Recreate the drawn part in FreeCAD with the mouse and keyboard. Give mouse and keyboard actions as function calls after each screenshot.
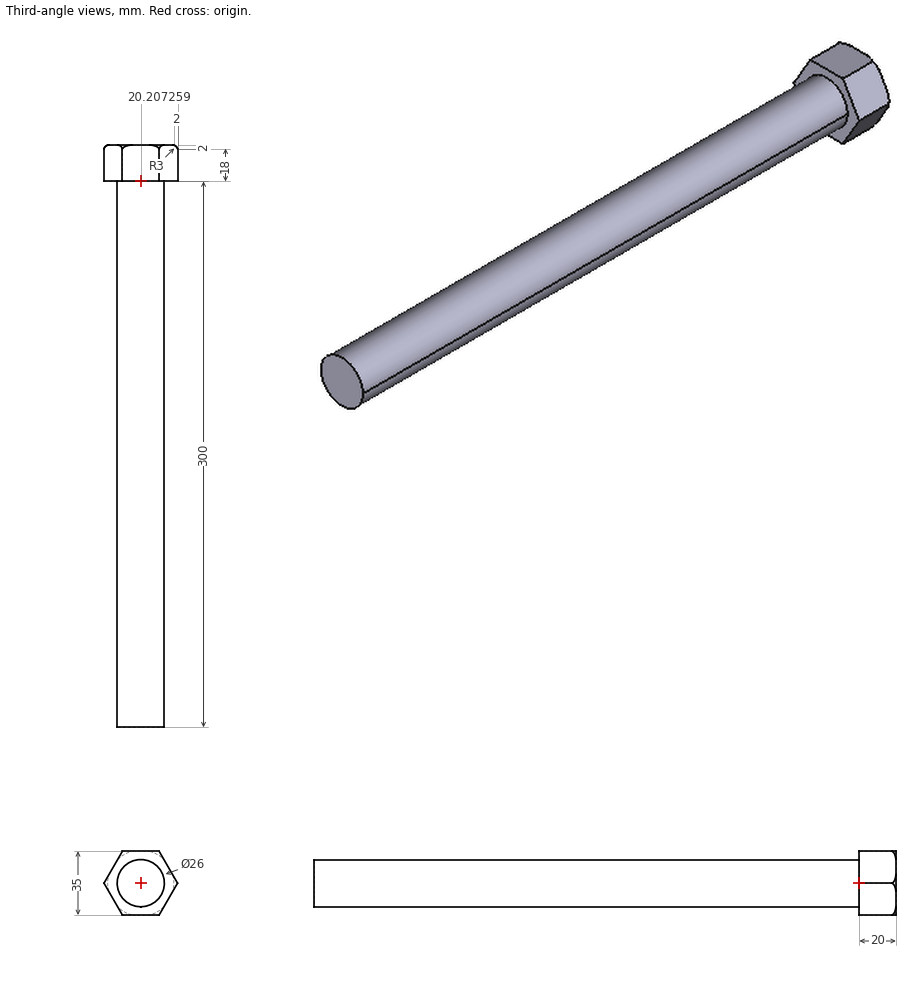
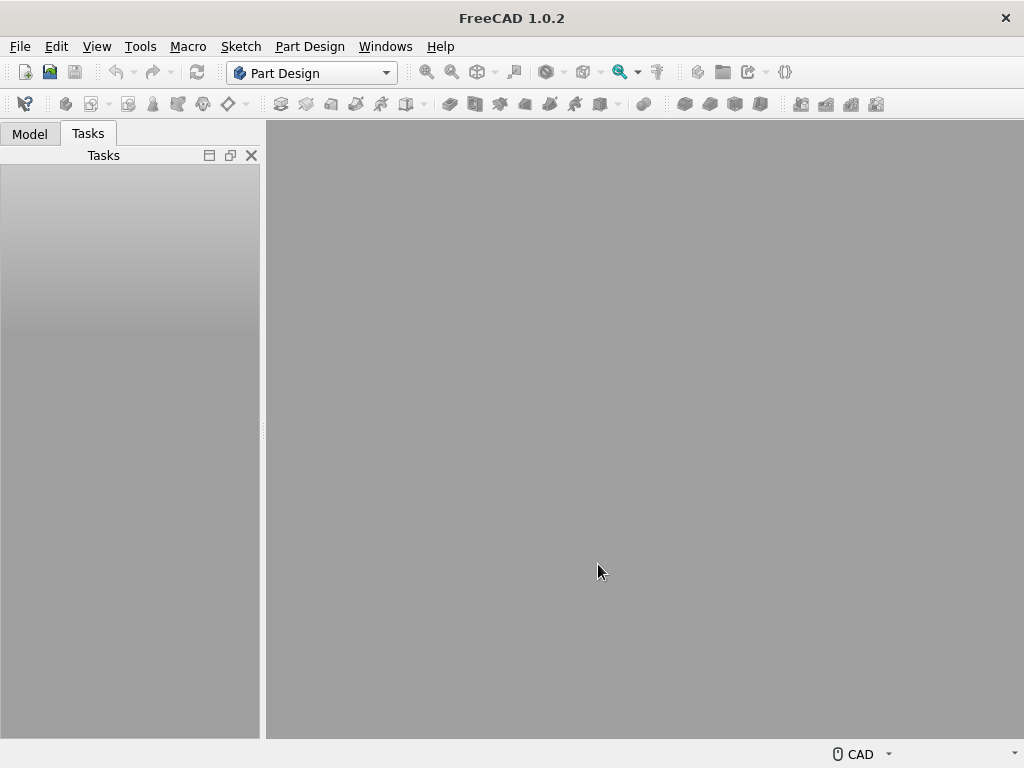
click(25, 72)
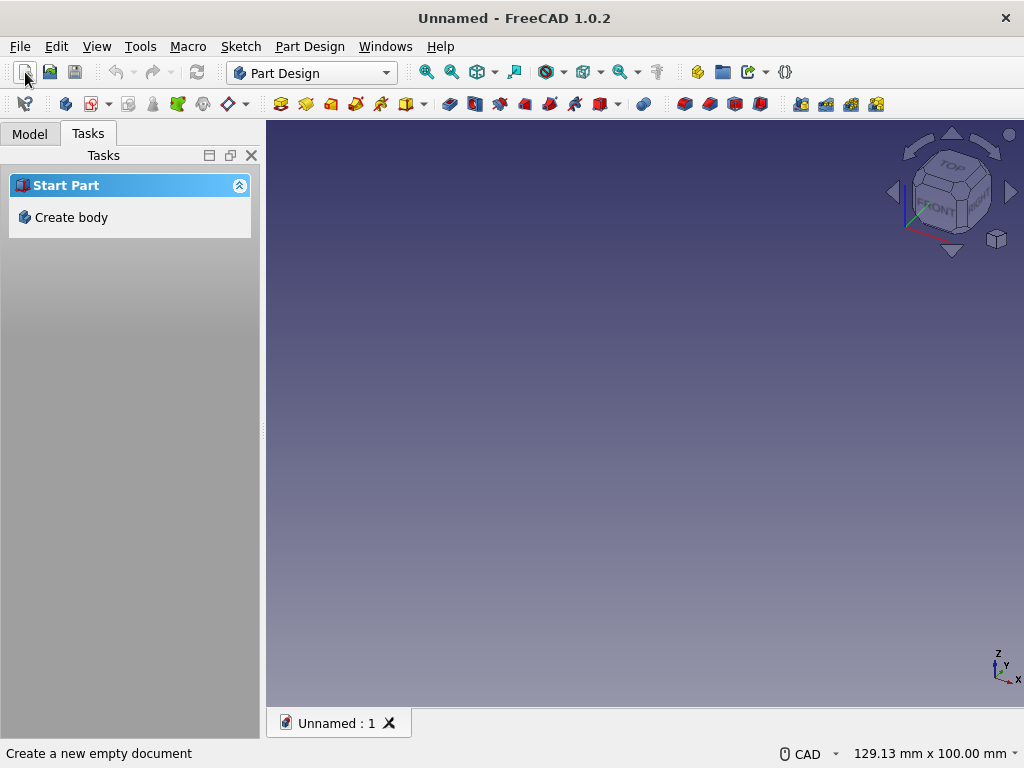
click(90, 104)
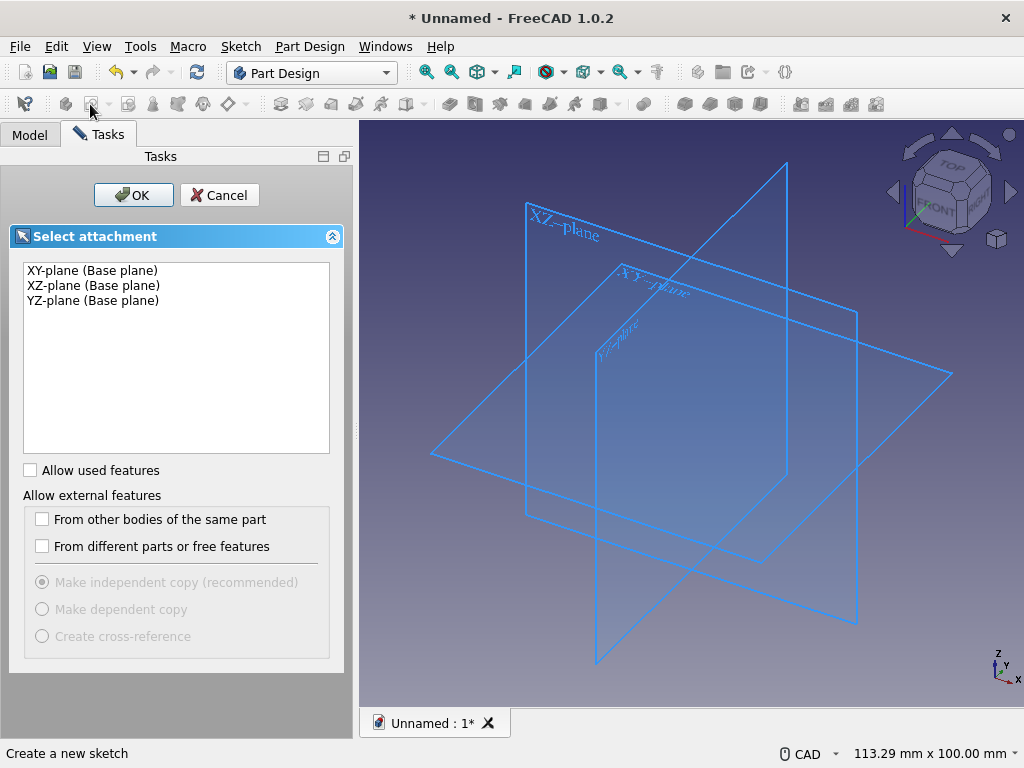
click(84, 286)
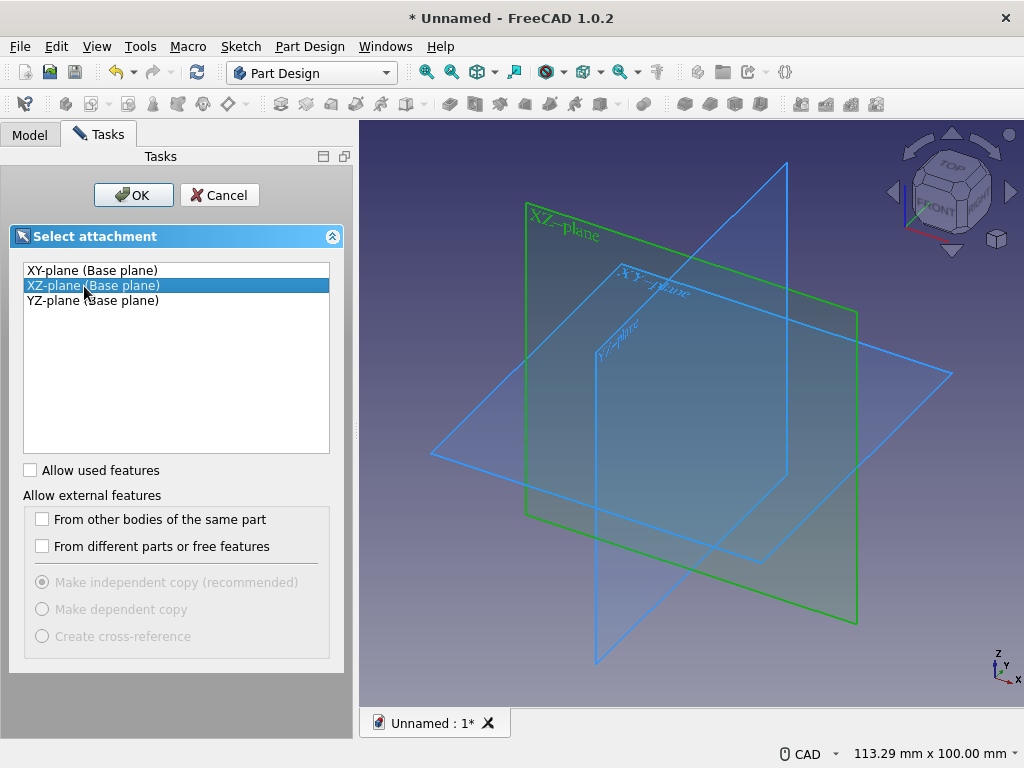
click(134, 195)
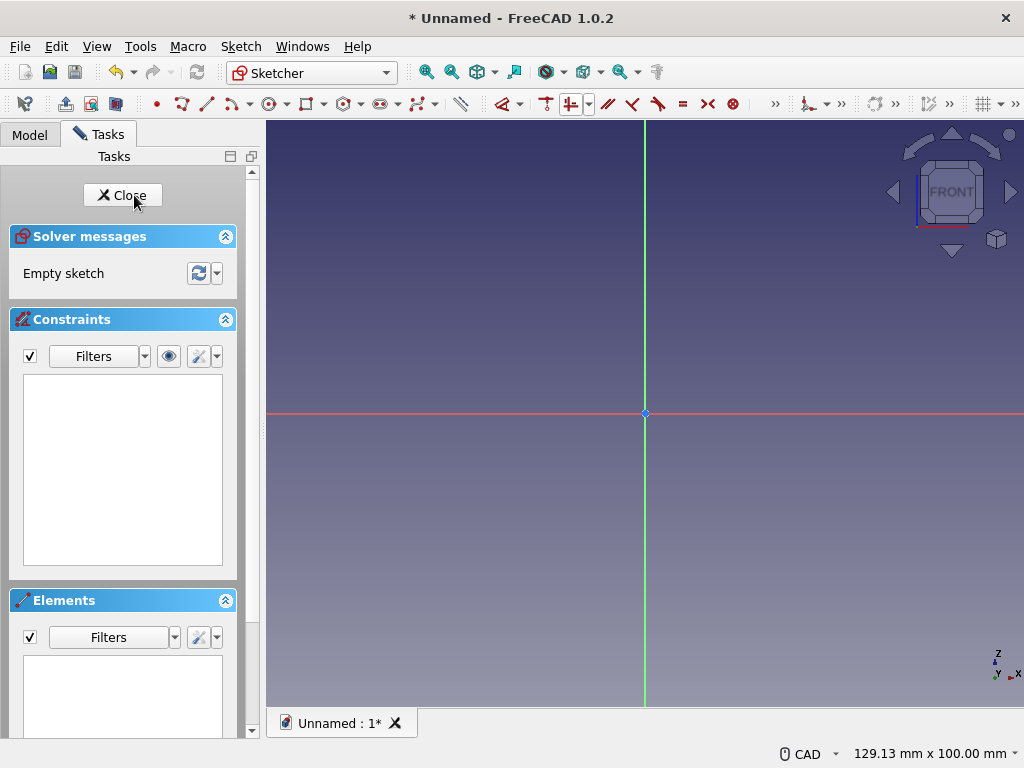
scroll(728, 414, up, 3)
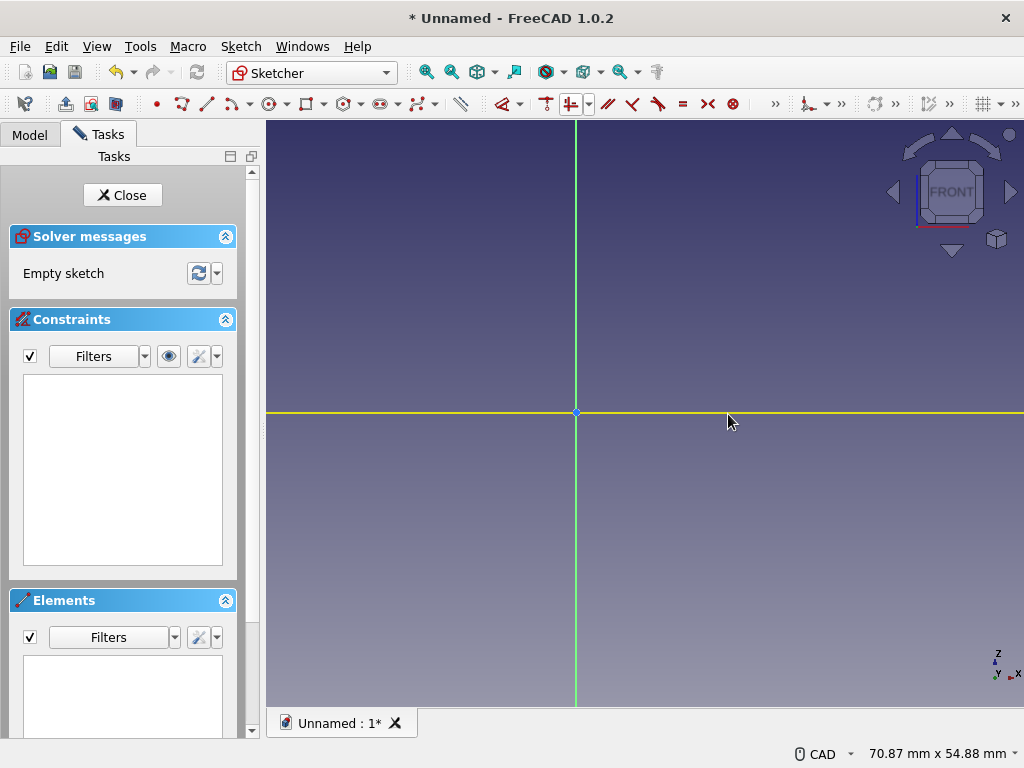
key(g)
key(p)
key(6)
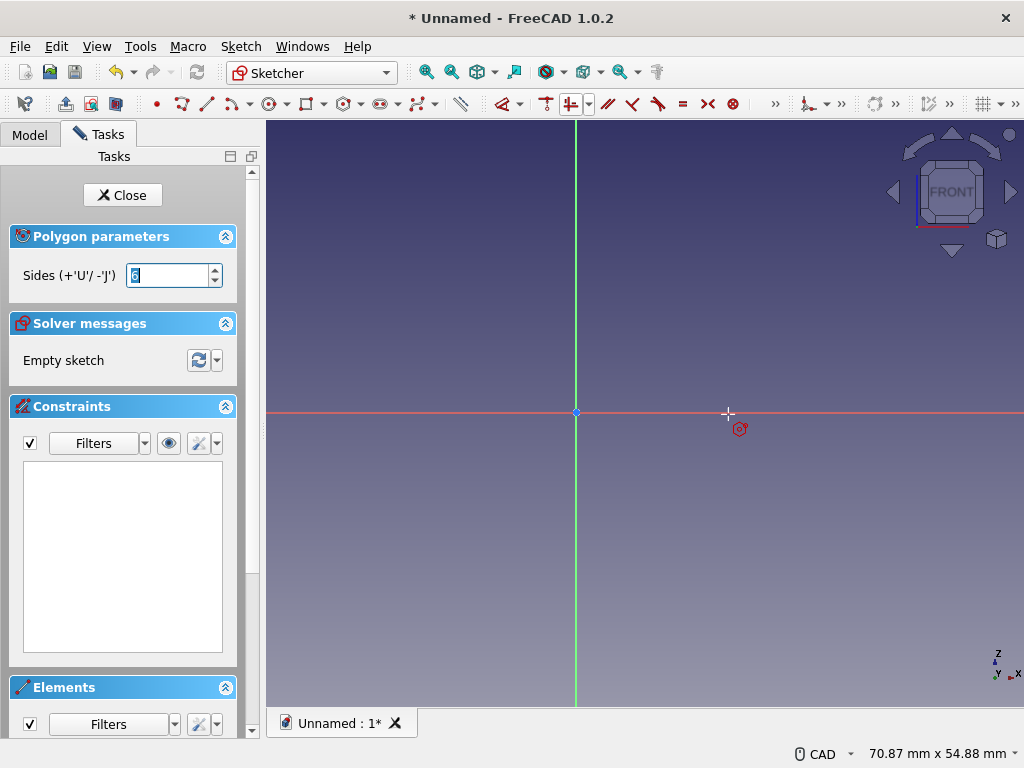
click(576, 413)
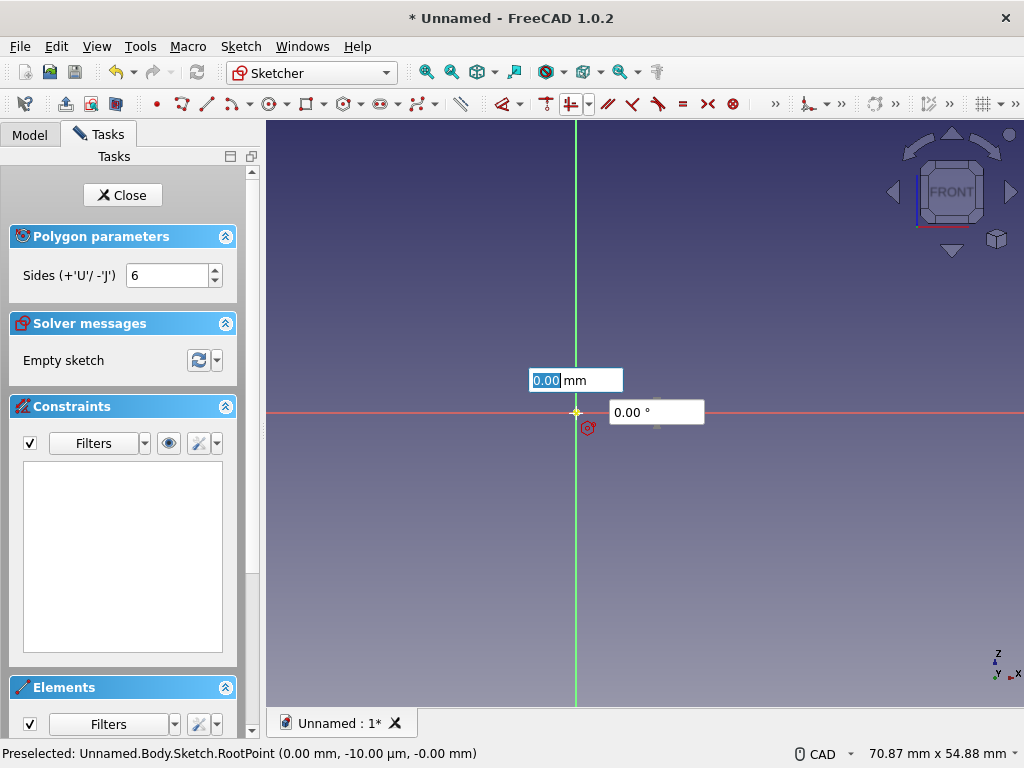
click(792, 413)
right_click(792, 413)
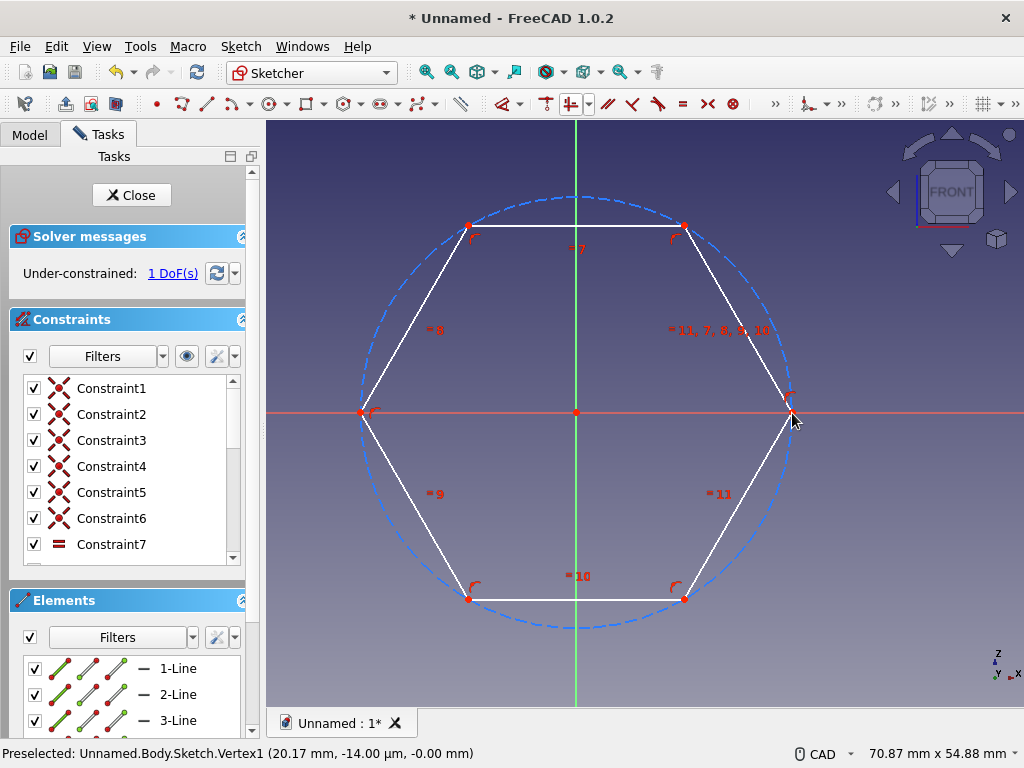
key(d)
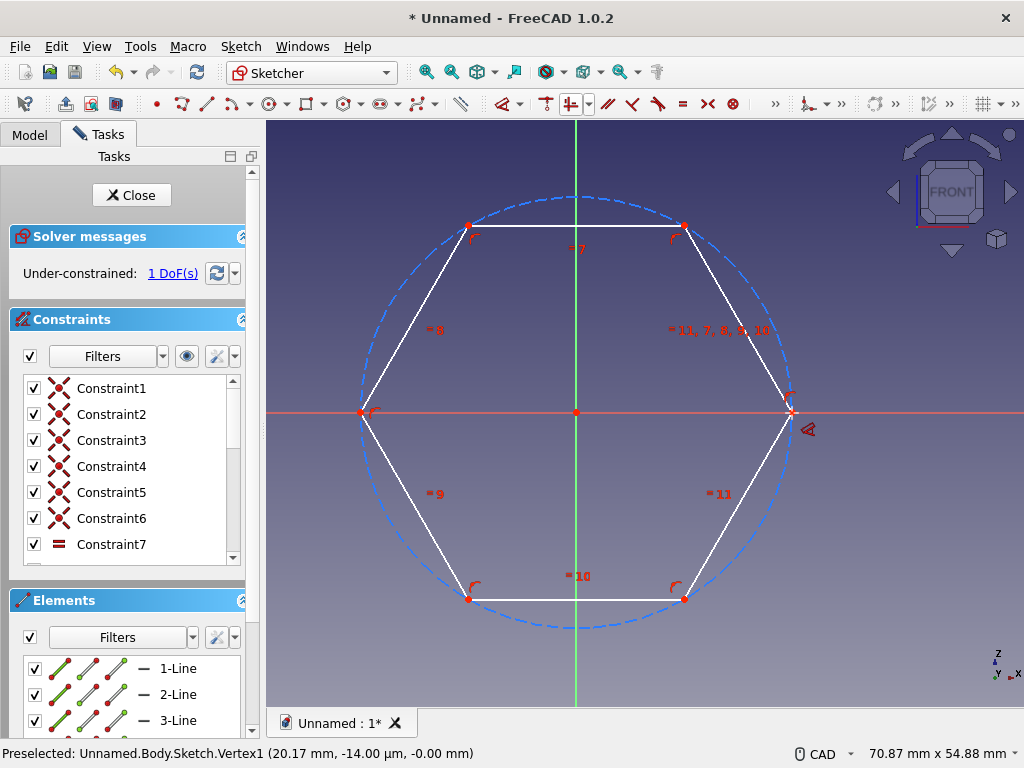
click(468, 600)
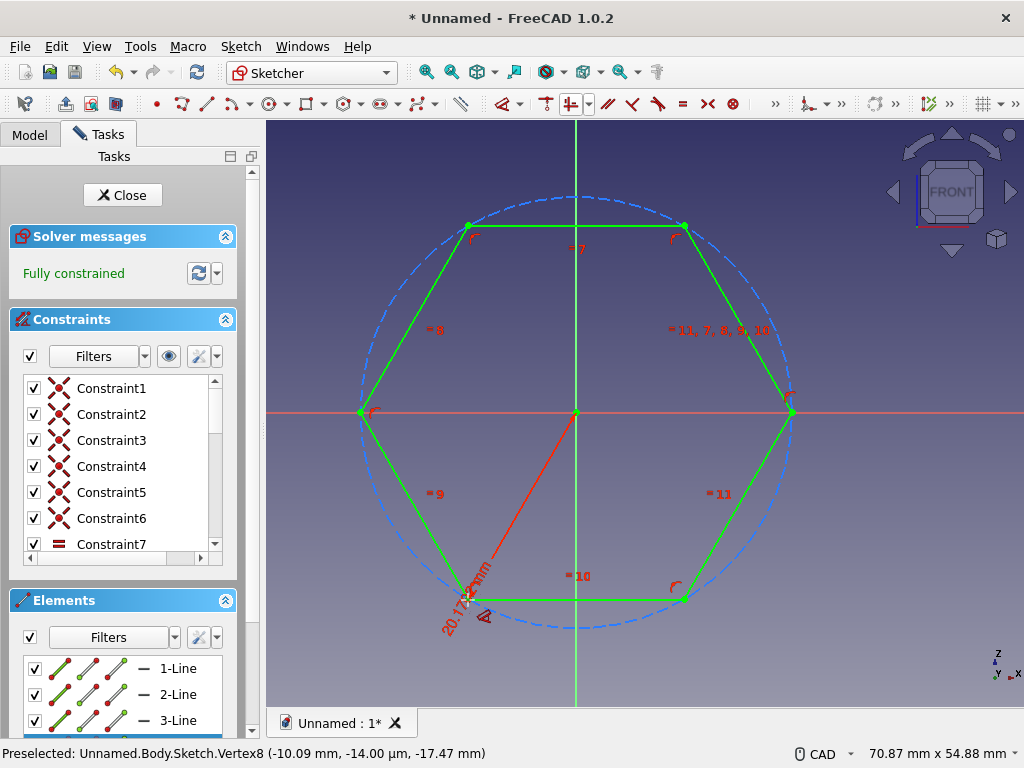
click(684, 226)
click(718, 327)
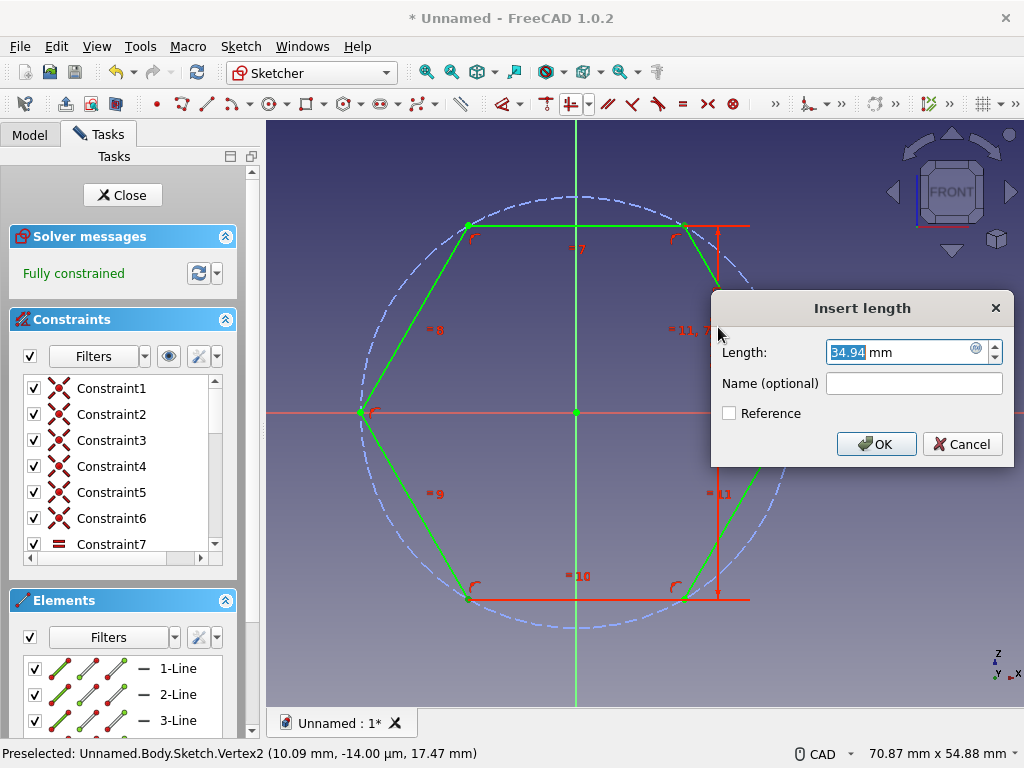
text(35)
key(Return)
key(Escape)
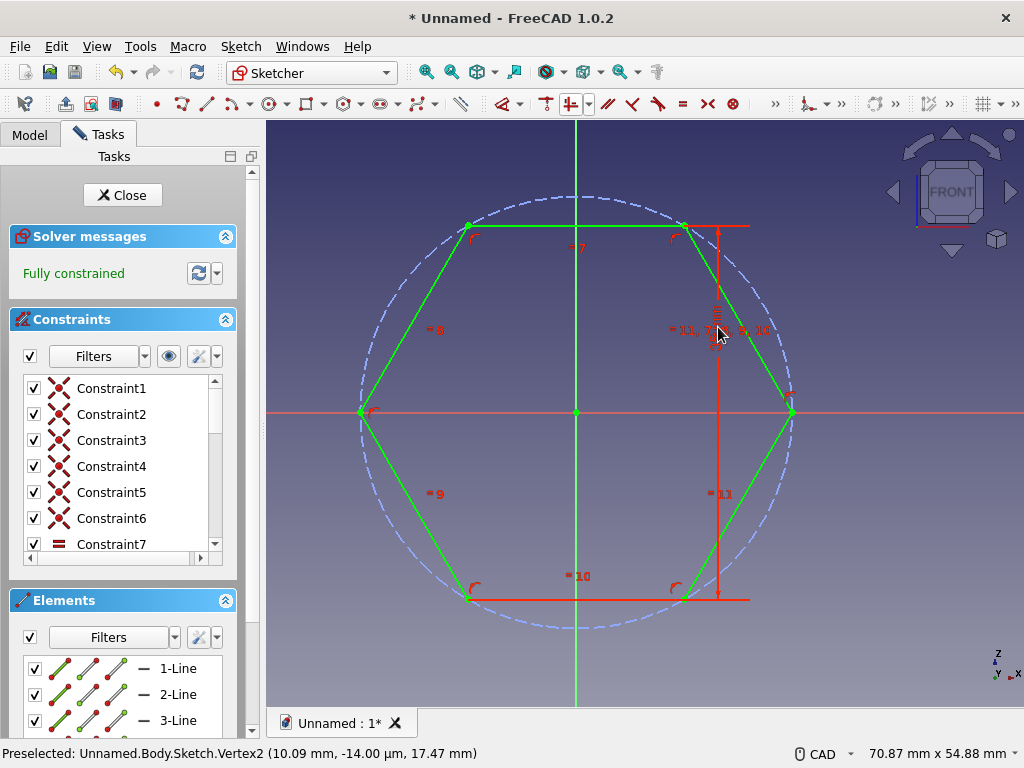
click(123, 195)